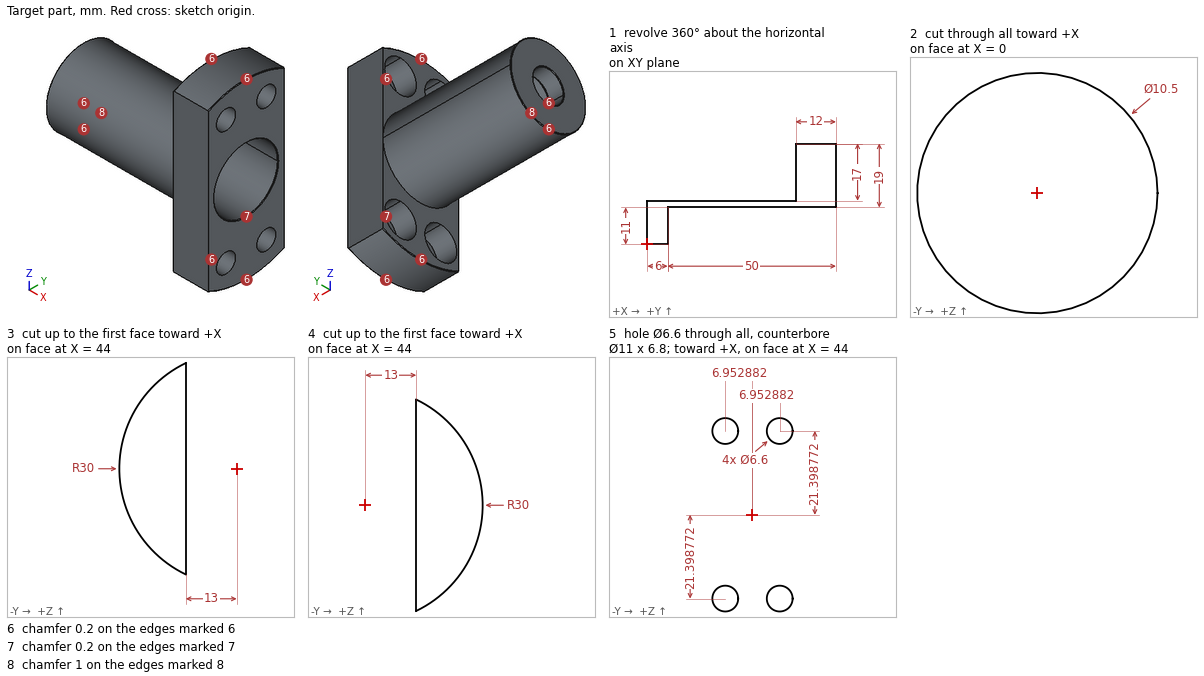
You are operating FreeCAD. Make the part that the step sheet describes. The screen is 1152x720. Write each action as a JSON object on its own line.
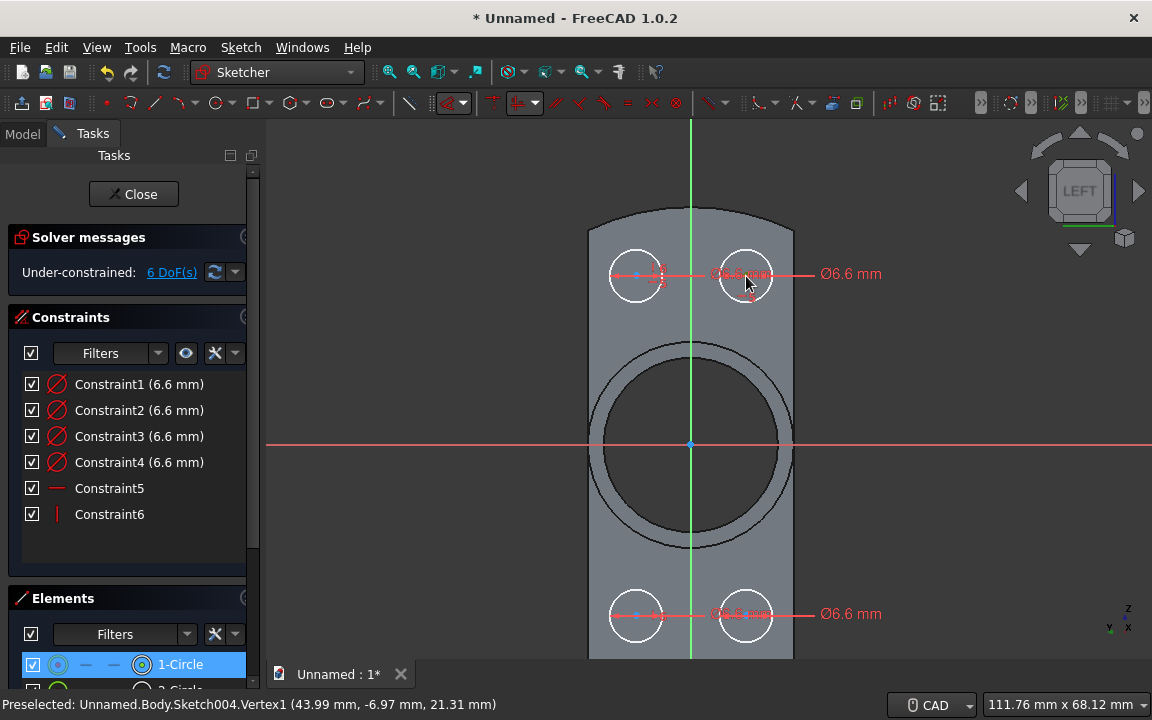
{"action": "left_click", "coordinate": [746, 616]}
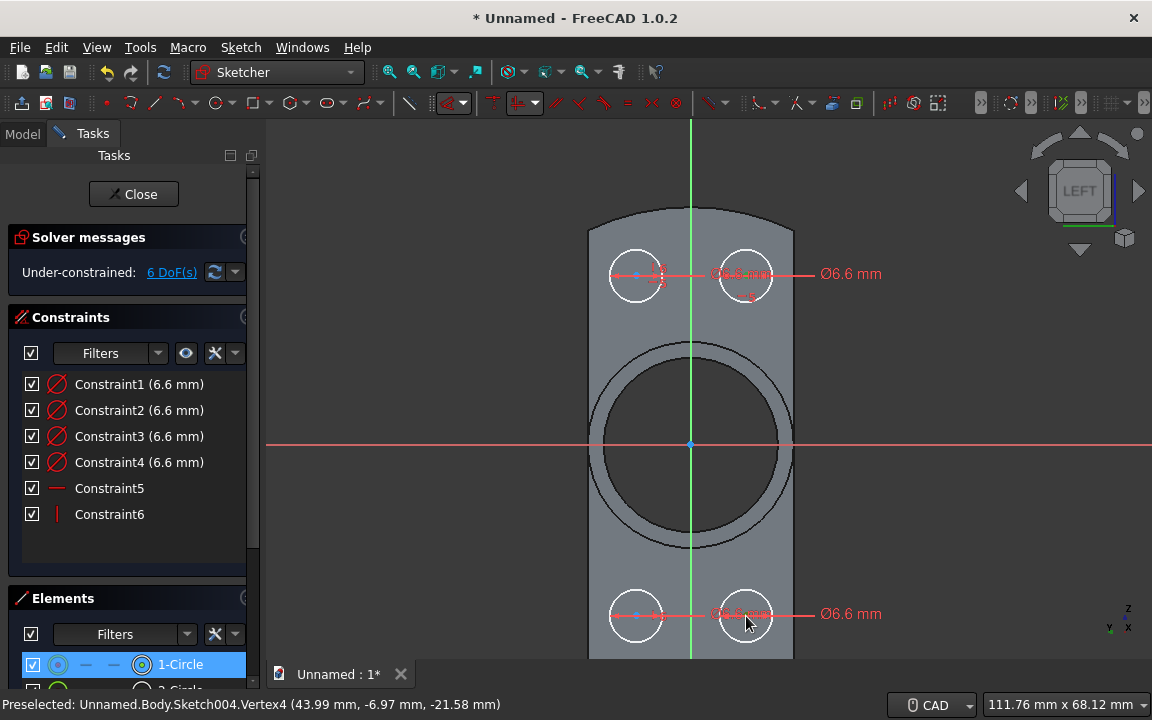
{"action": "key", "text": "v"}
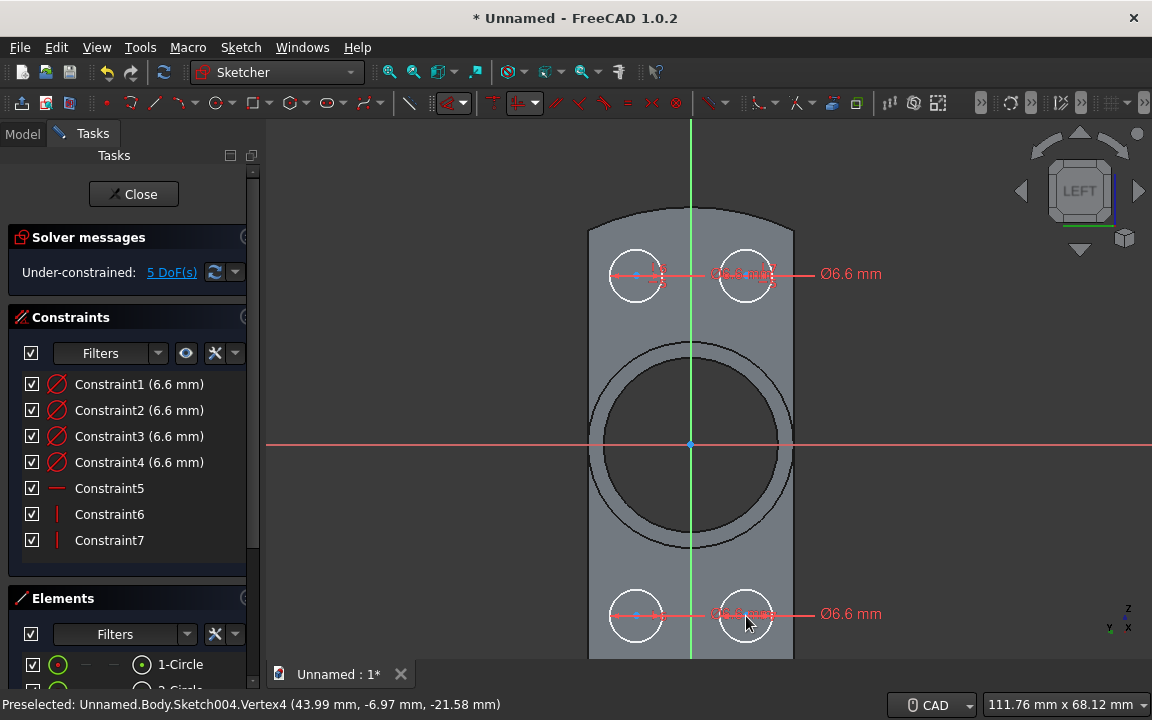
{"action": "left_click", "coordinate": [636, 616]}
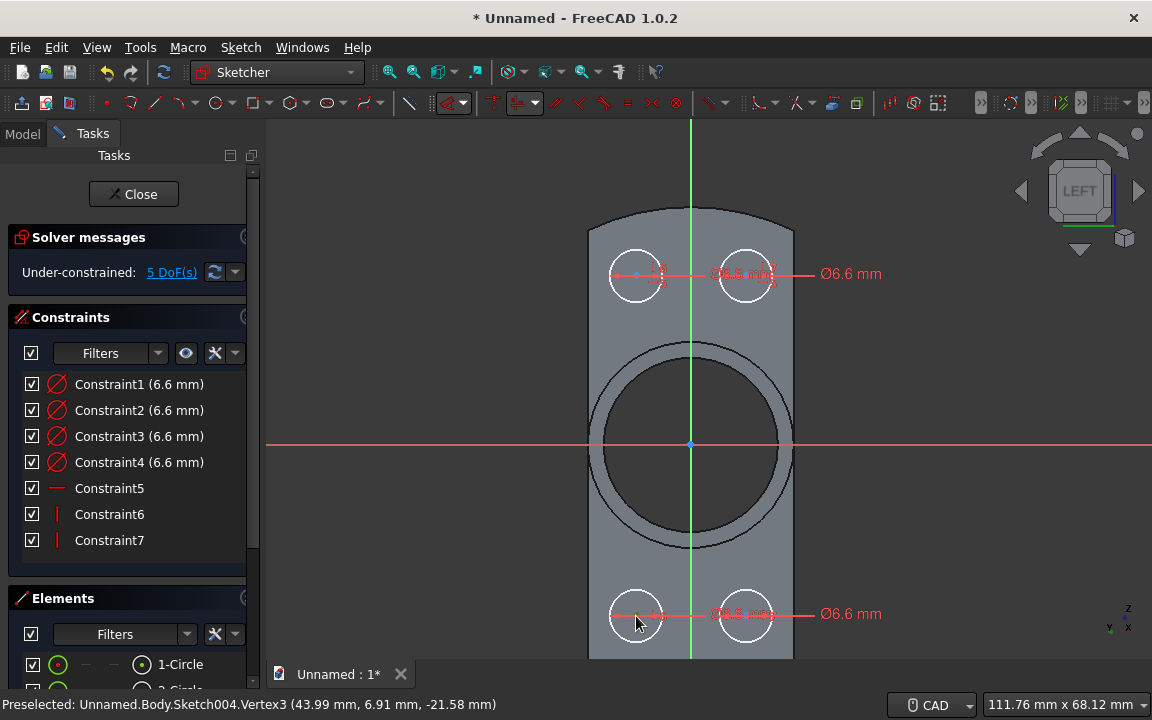
{"action": "left_click", "coordinate": [746, 616]}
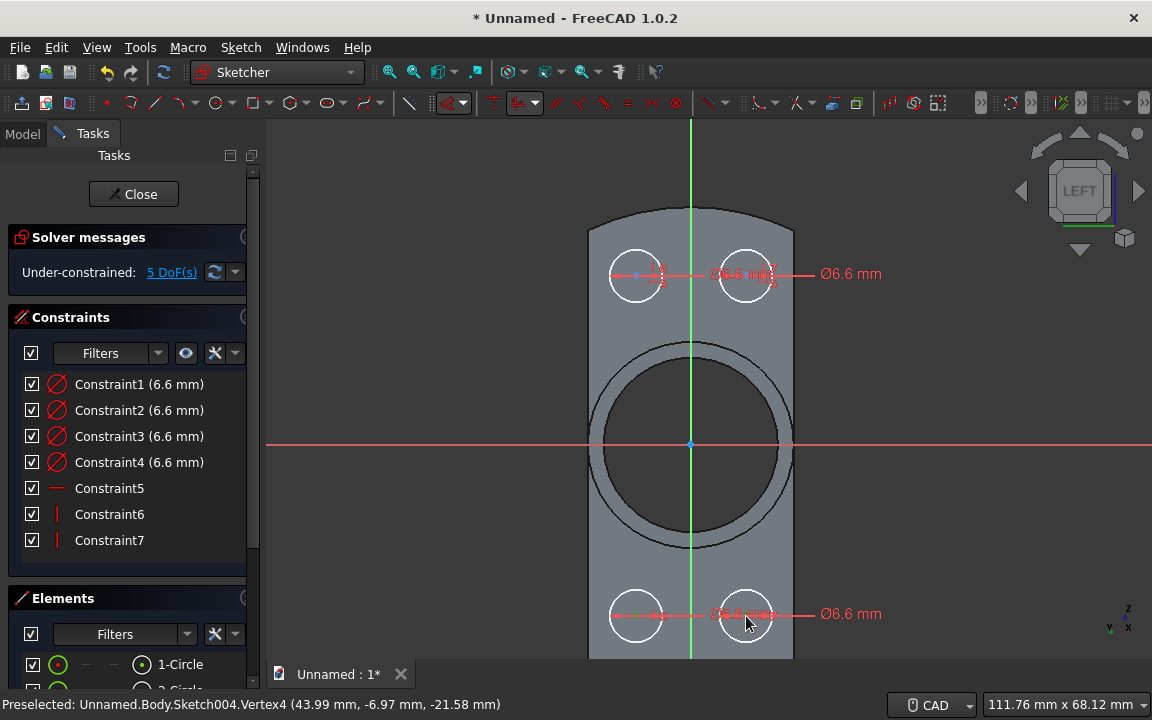
{"action": "key", "text": "h"}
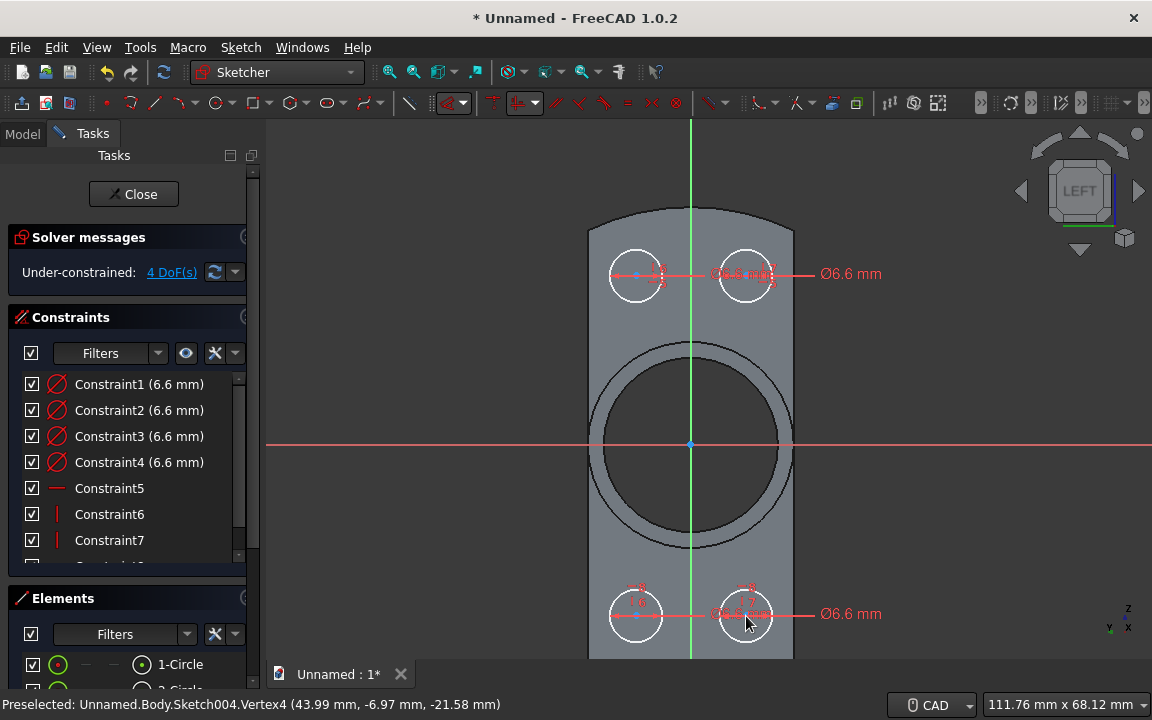
{"action": "left_click", "coordinate": [746, 276]}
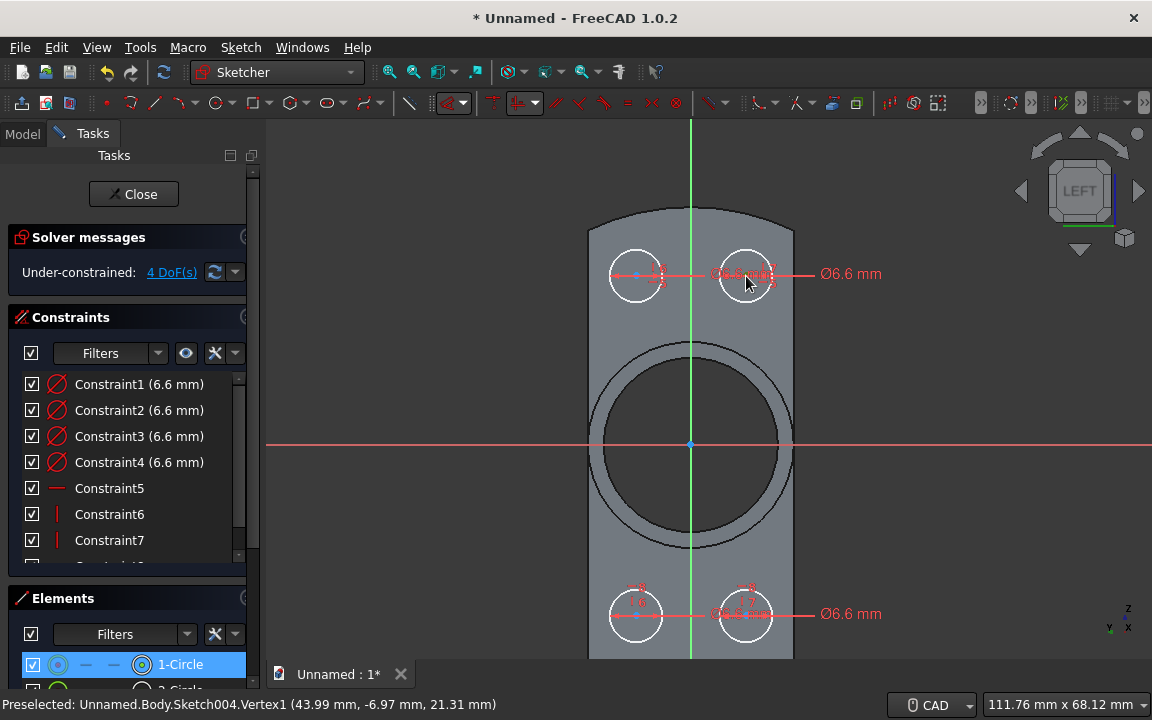
{"action": "key", "text": "l"}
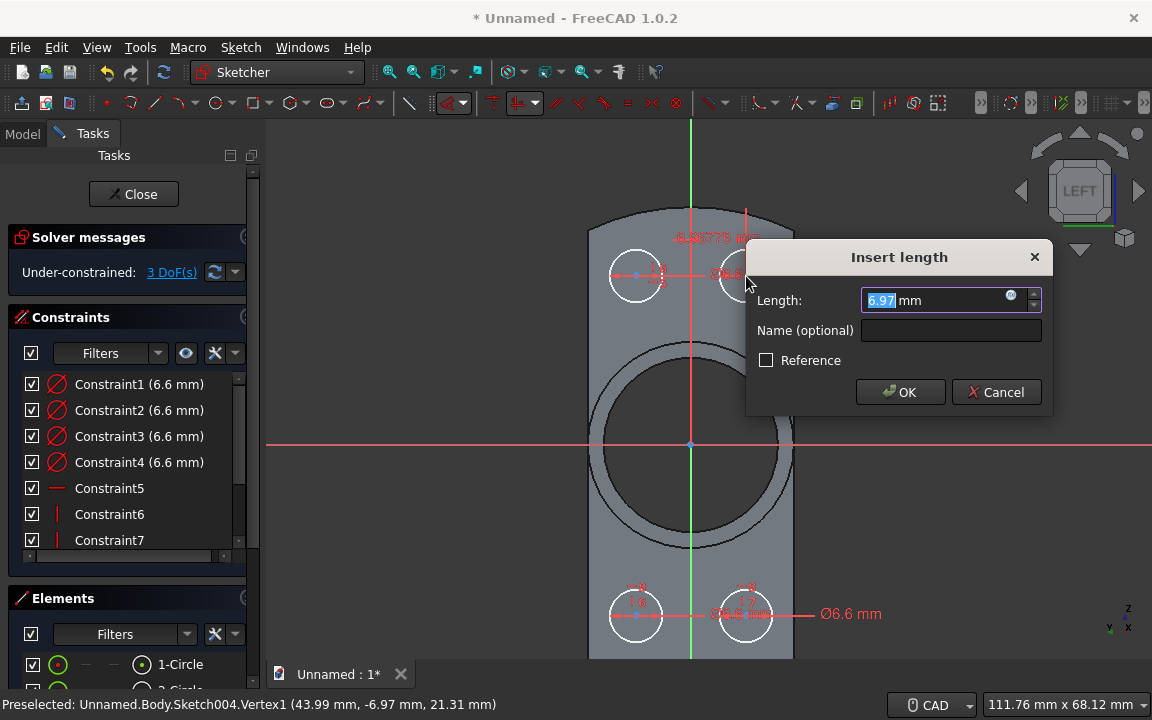
{"action": "type", "text": "6.952882"}
{"action": "key", "text": "Return"}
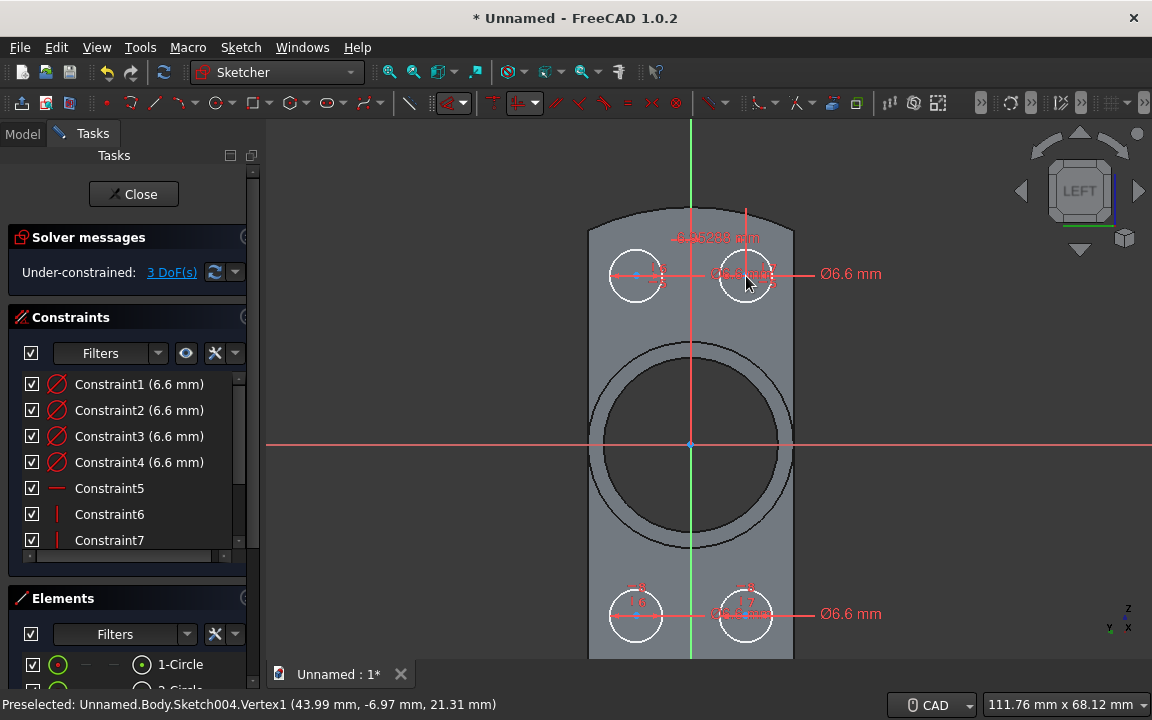
{"action": "left_click", "coordinate": [636, 276]}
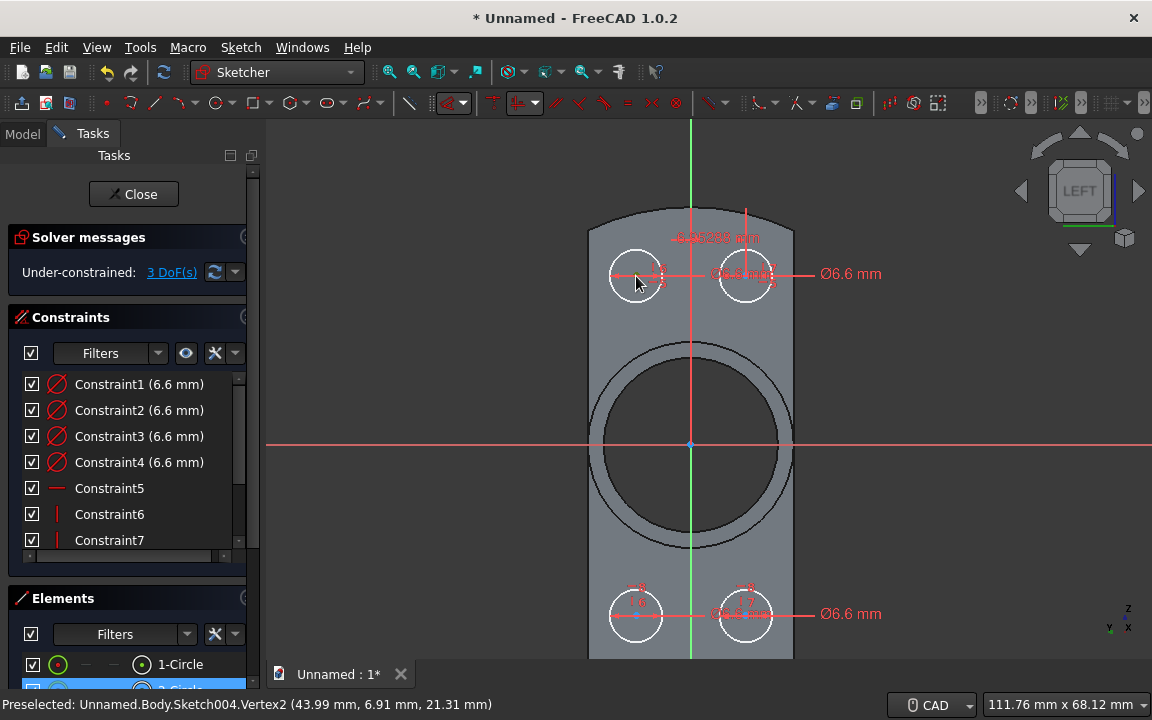
{"action": "left_click", "coordinate": [466, 104]}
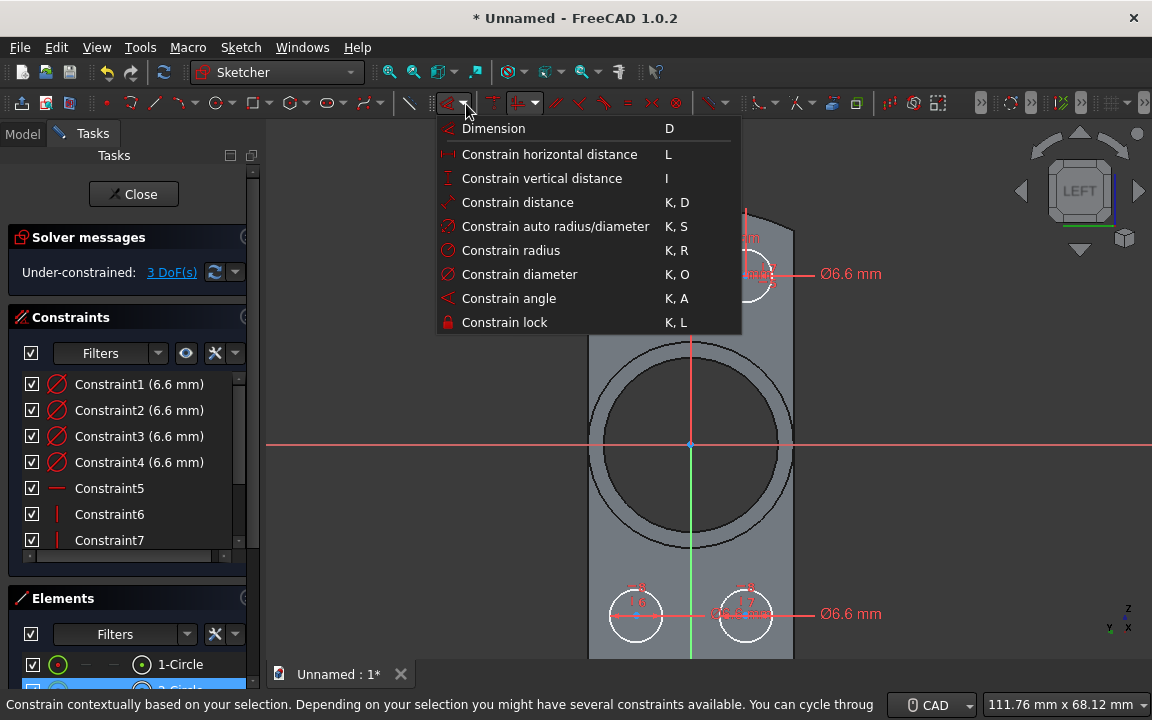
{"action": "left_click", "coordinate": [589, 154]}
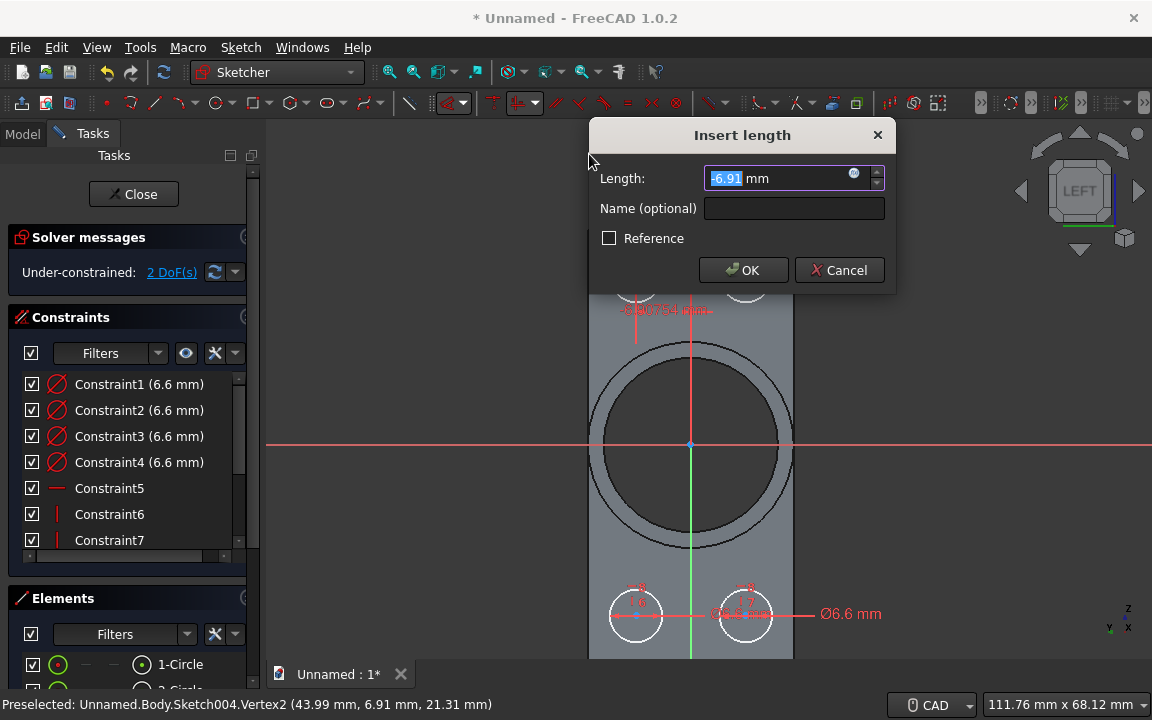
{"action": "type", "text": "-6.952882"}
{"action": "key", "text": "Return"}